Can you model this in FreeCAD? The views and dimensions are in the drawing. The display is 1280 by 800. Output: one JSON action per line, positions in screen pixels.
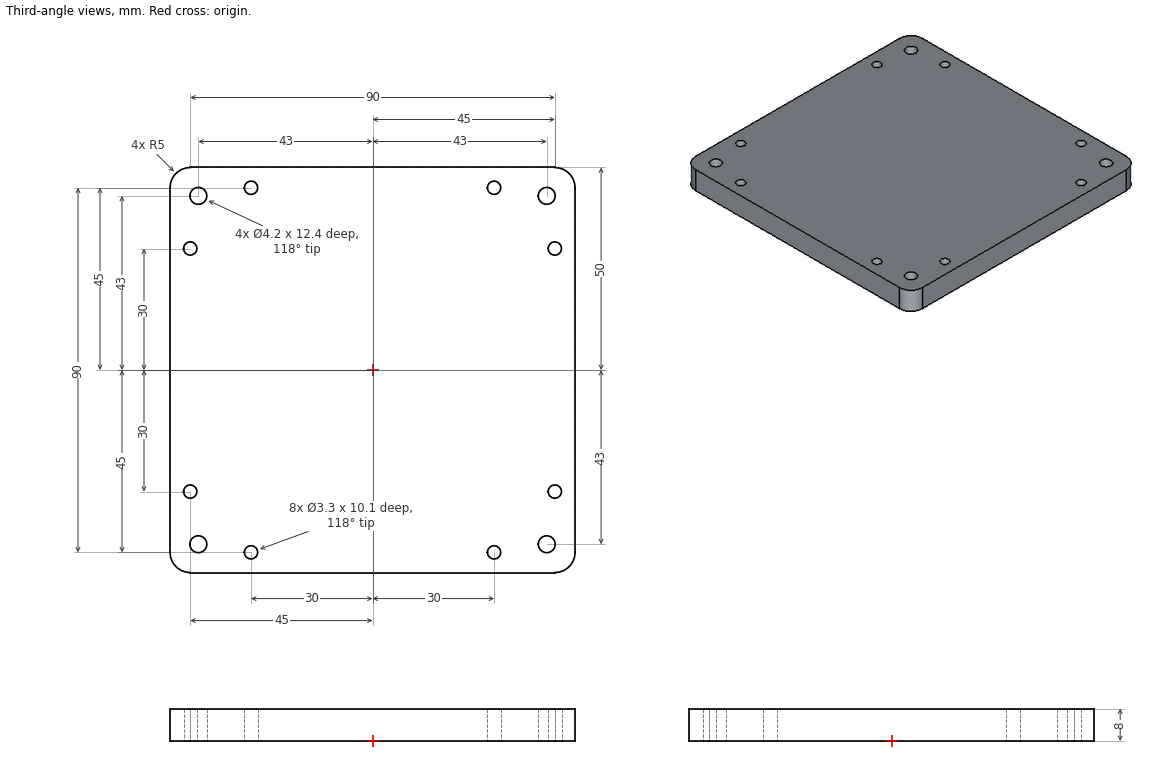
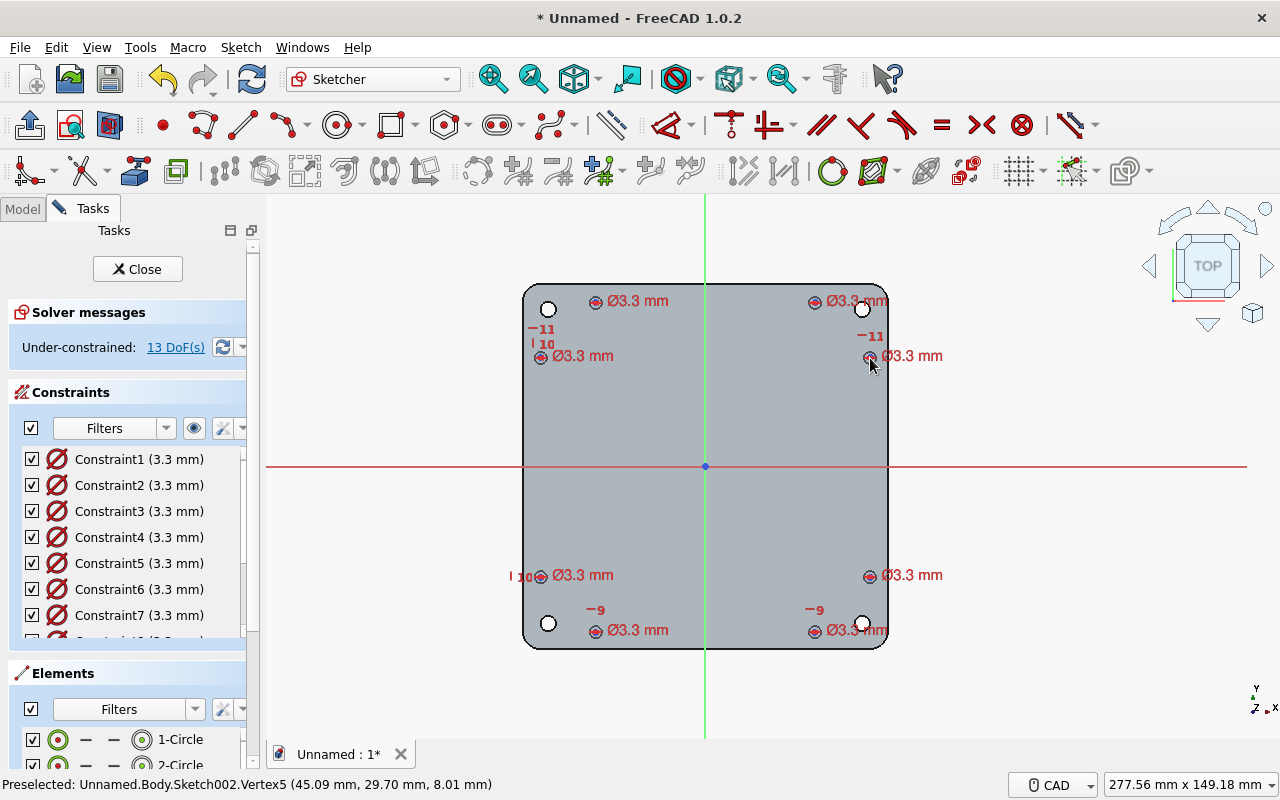
{"action": "left_click", "coordinate": [870, 358]}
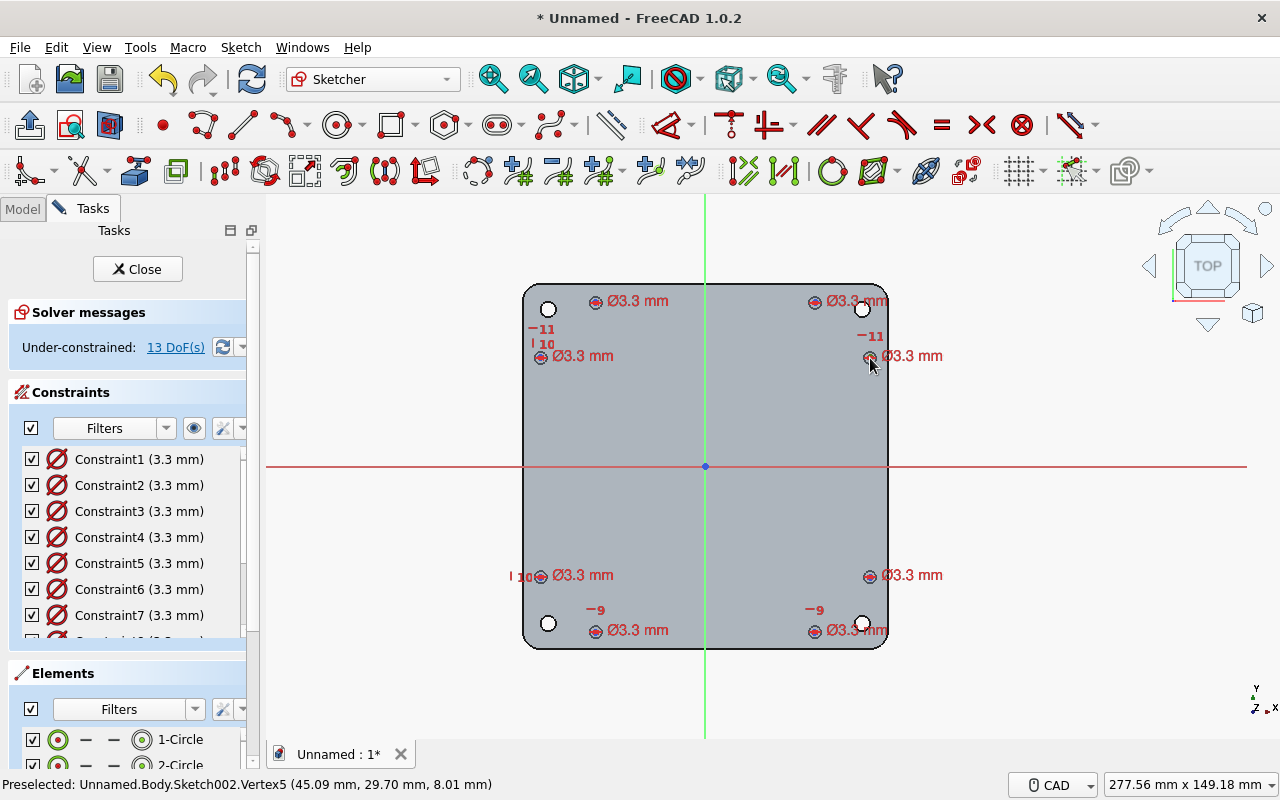
{"action": "left_click", "coordinate": [870, 577]}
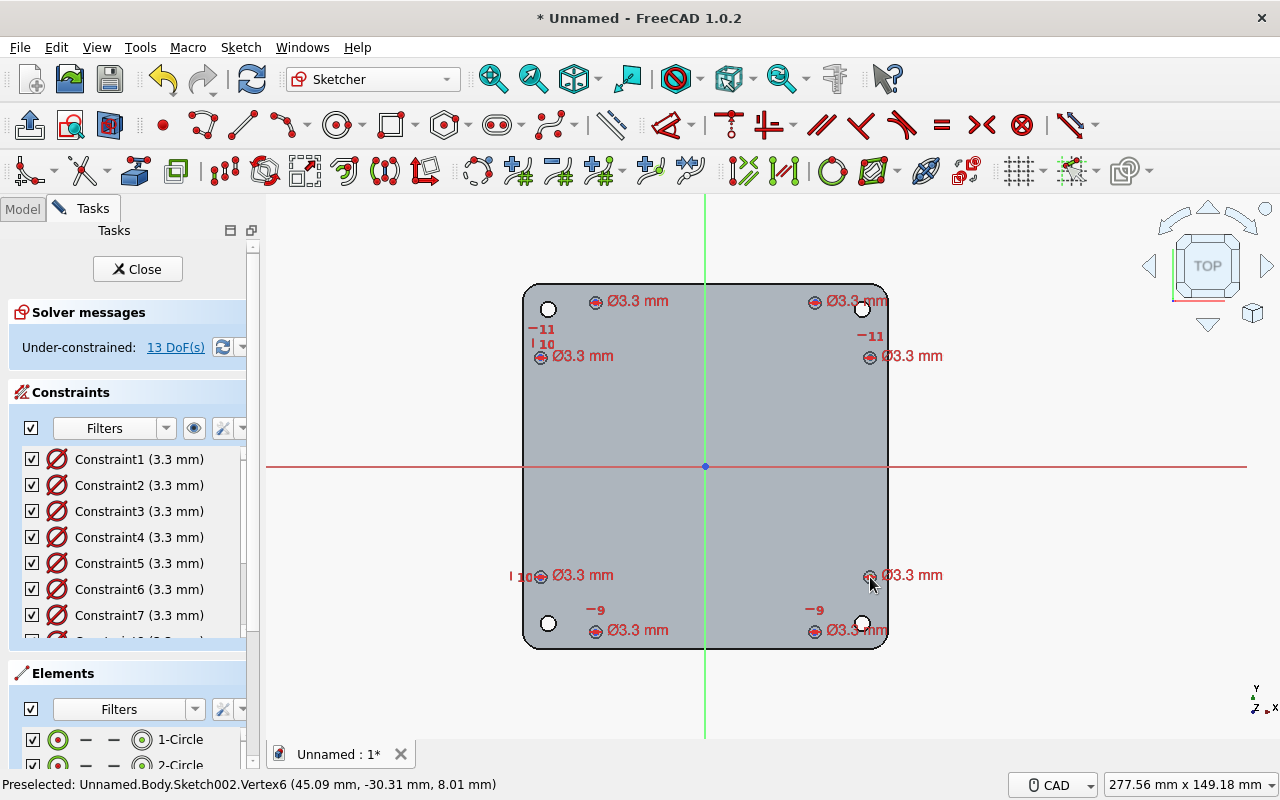
{"action": "key", "text": "v"}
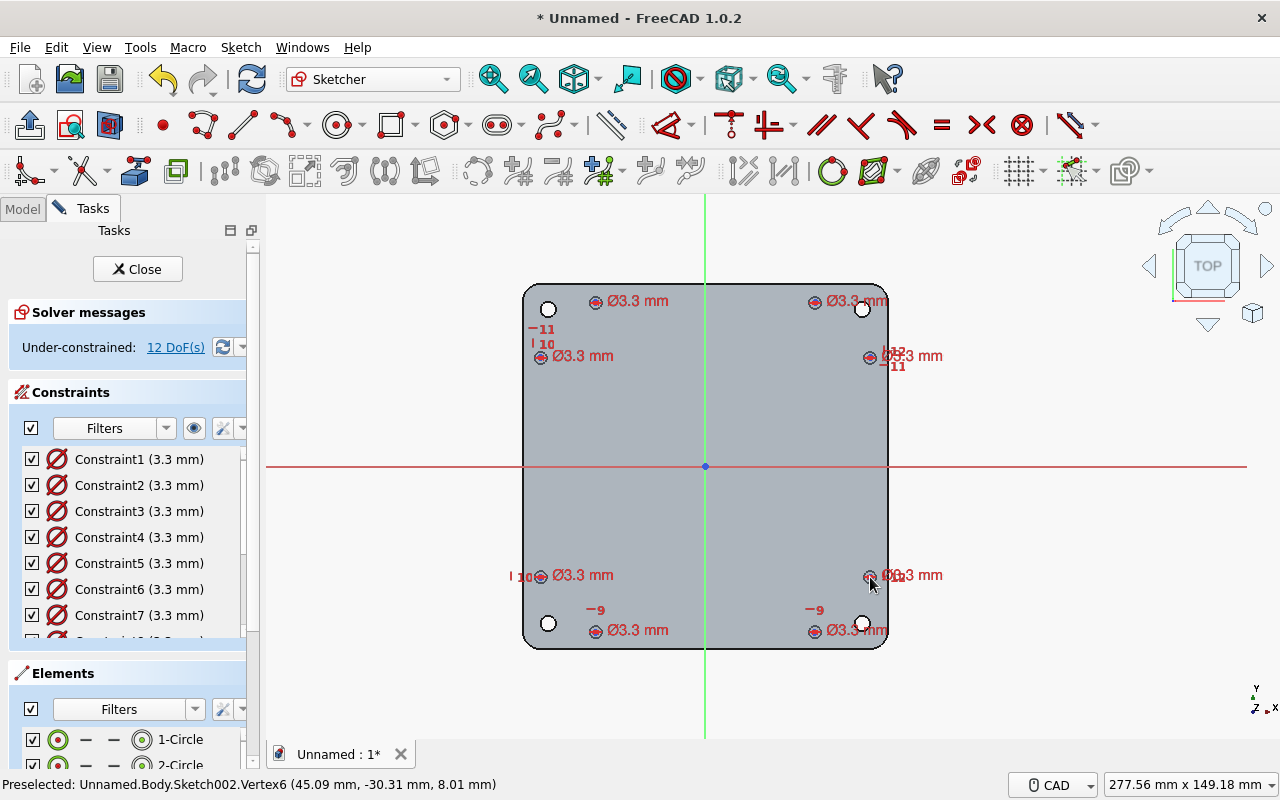
{"action": "left_click", "coordinate": [541, 577]}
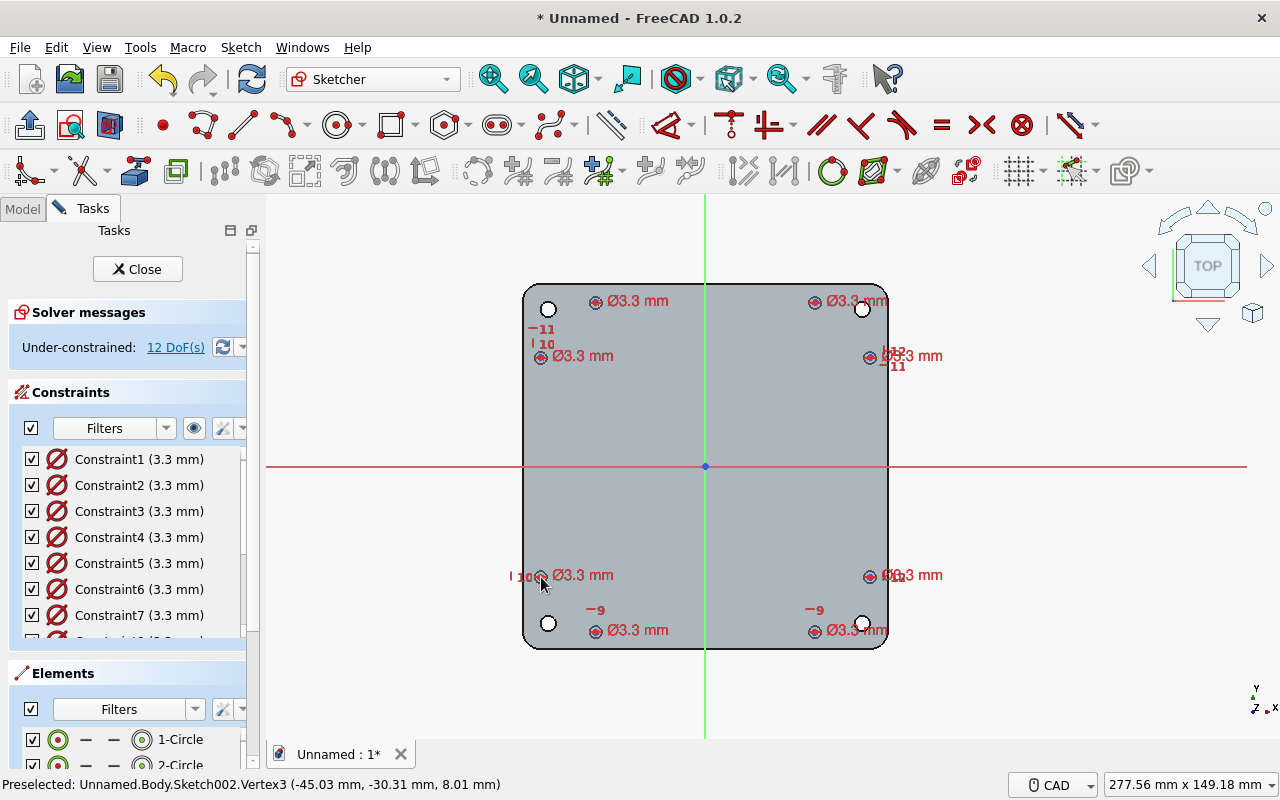
{"action": "left_click", "coordinate": [870, 577]}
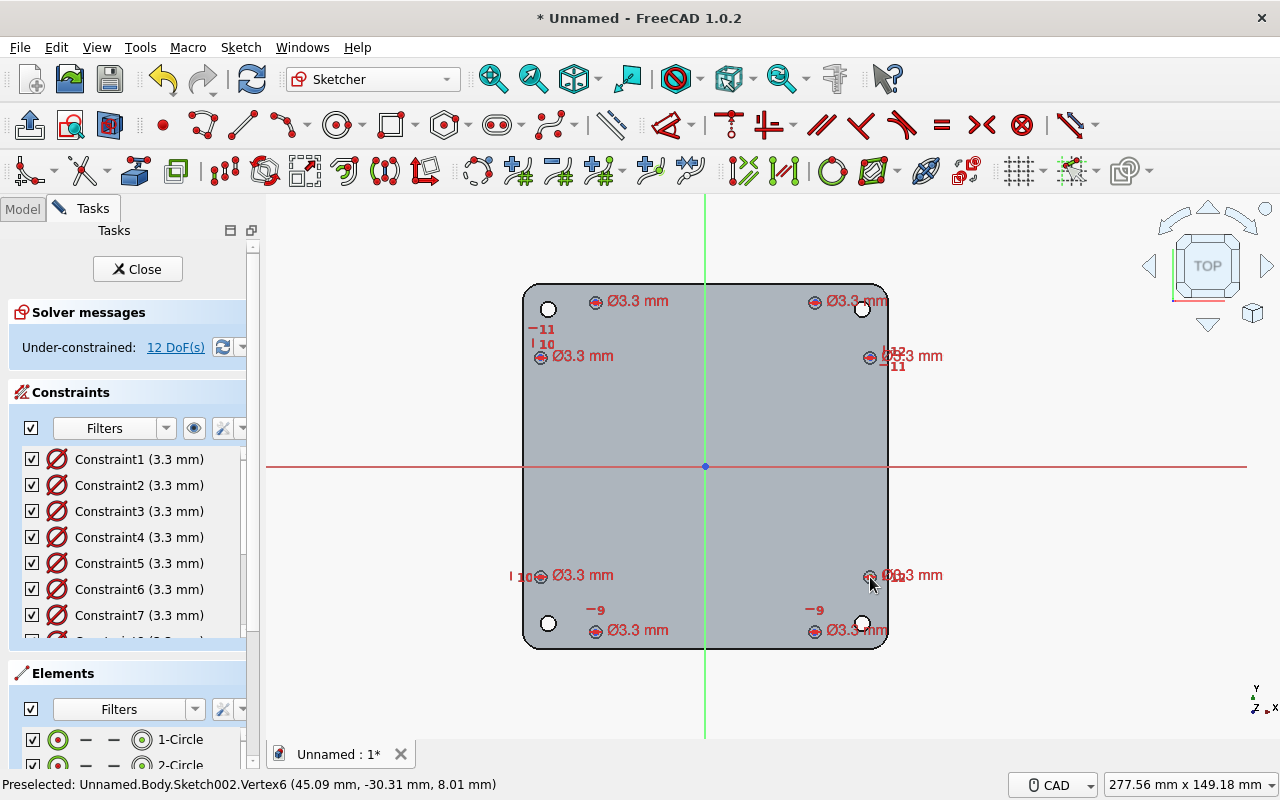
{"action": "key", "text": "h"}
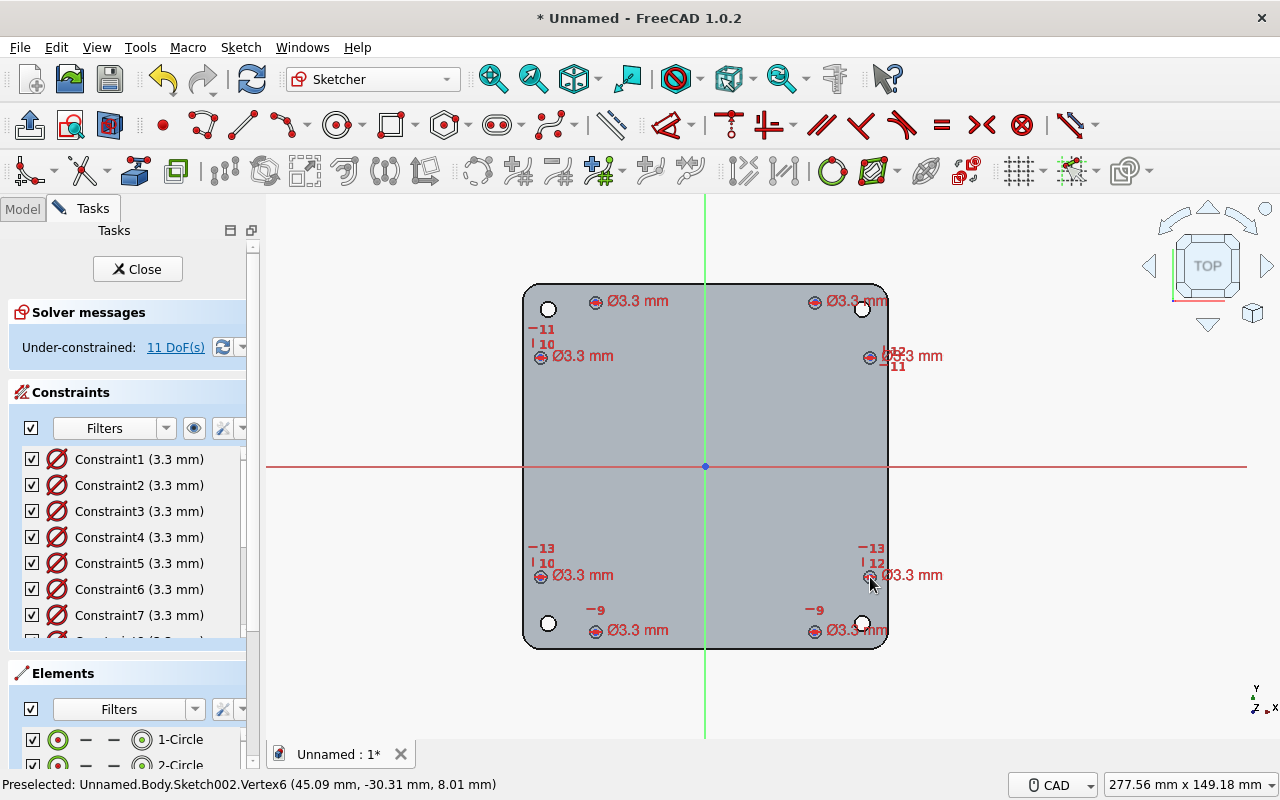
{"action": "left_click", "coordinate": [596, 632]}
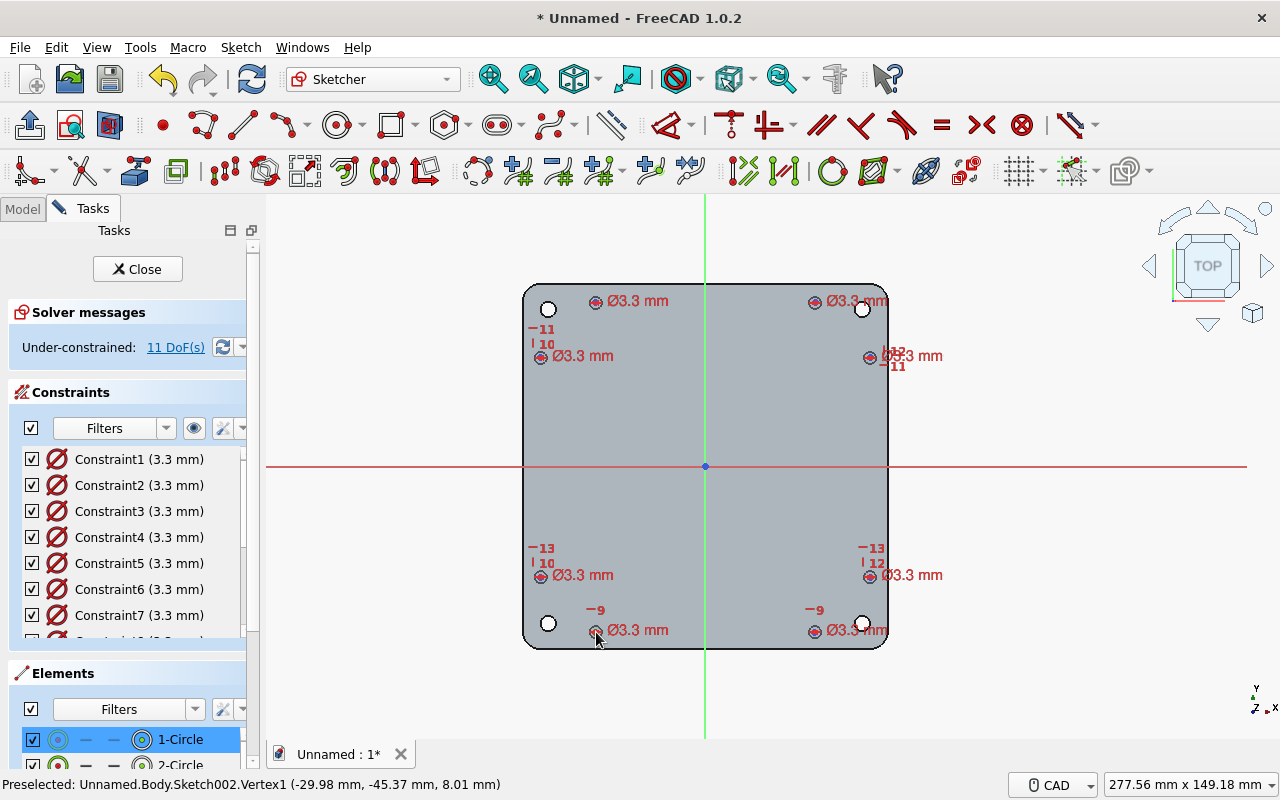
{"action": "left_click", "coordinate": [596, 303]}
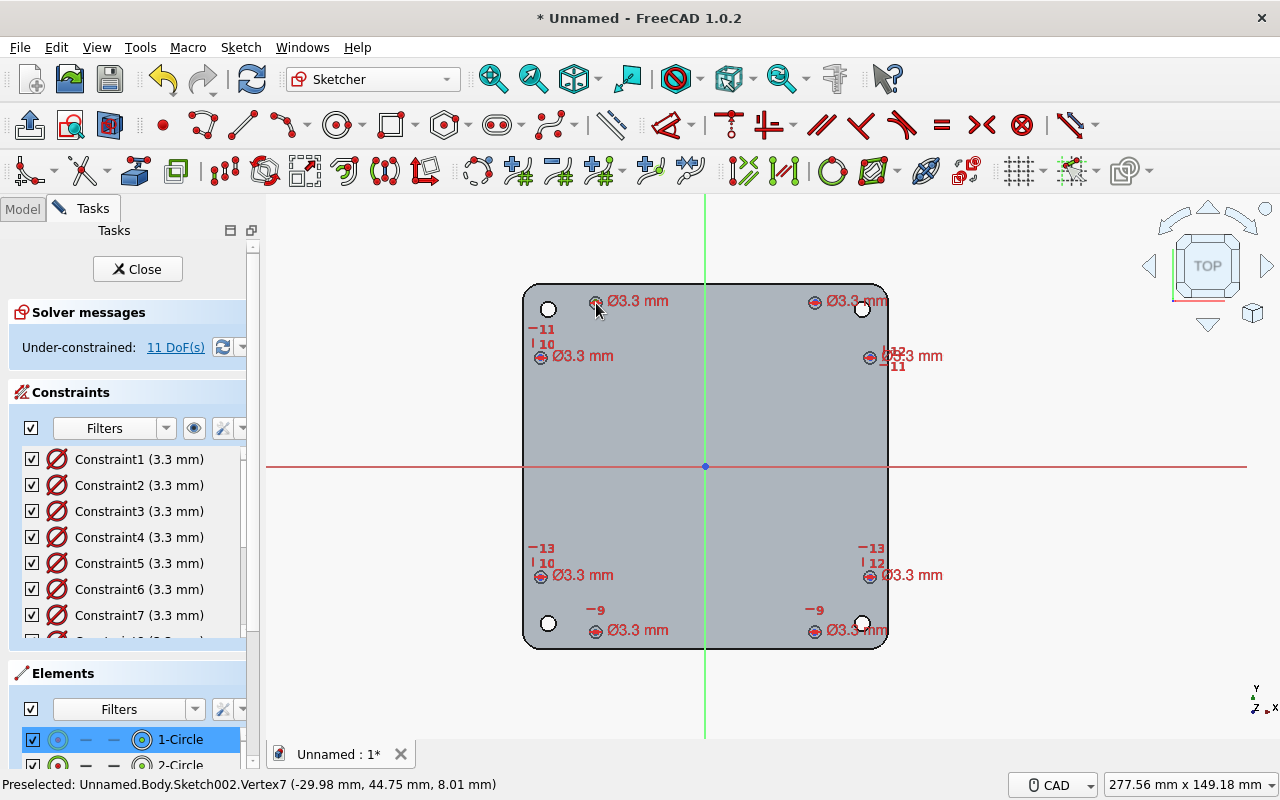
{"action": "key", "text": "v"}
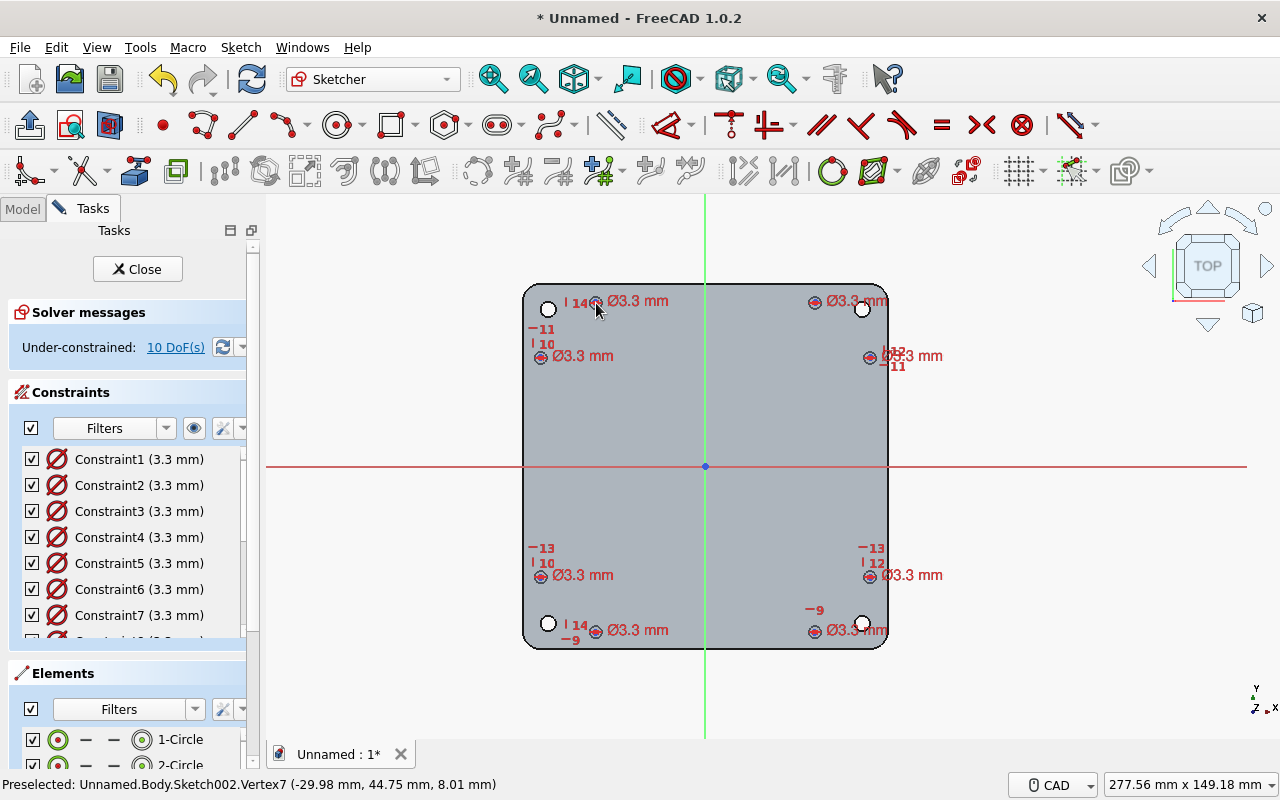
{"action": "left_click", "coordinate": [815, 632]}